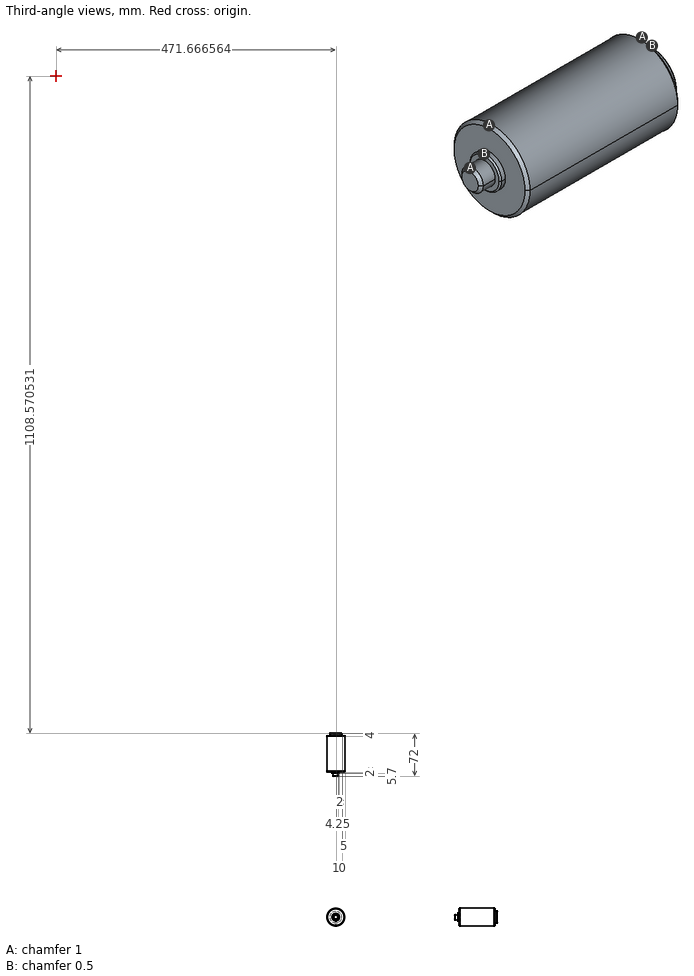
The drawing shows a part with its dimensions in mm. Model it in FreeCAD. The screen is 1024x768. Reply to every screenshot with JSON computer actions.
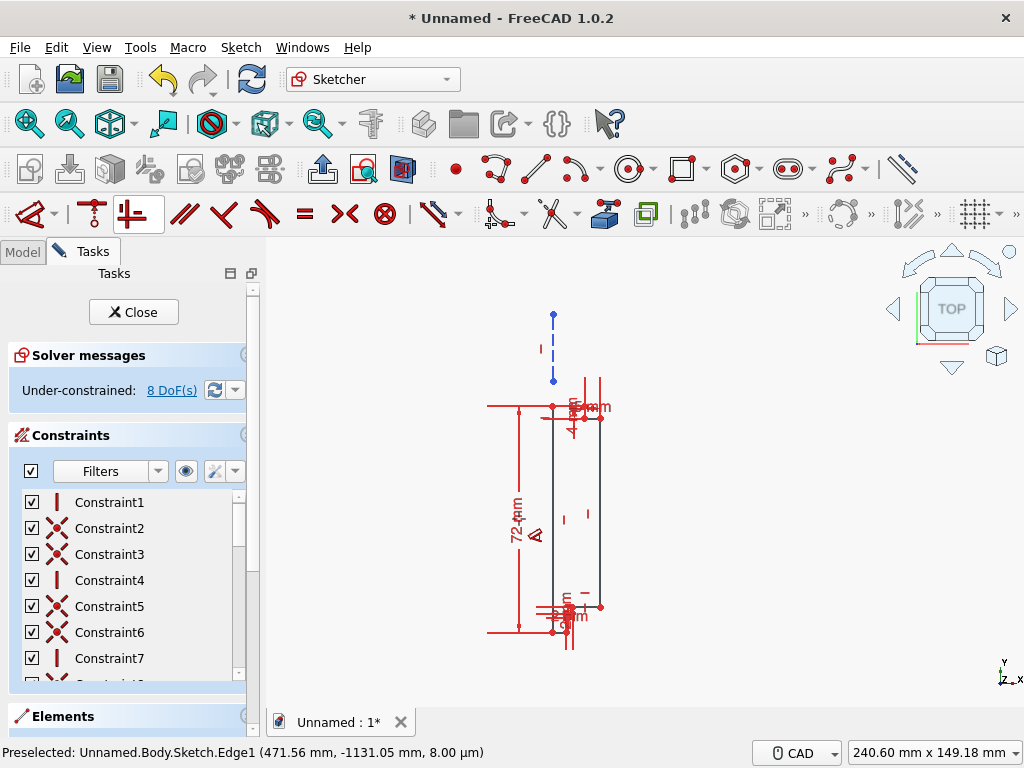
{"action": "scroll", "coordinate": [575, 406], "scroll_direction": "up", "scroll_amount": 2}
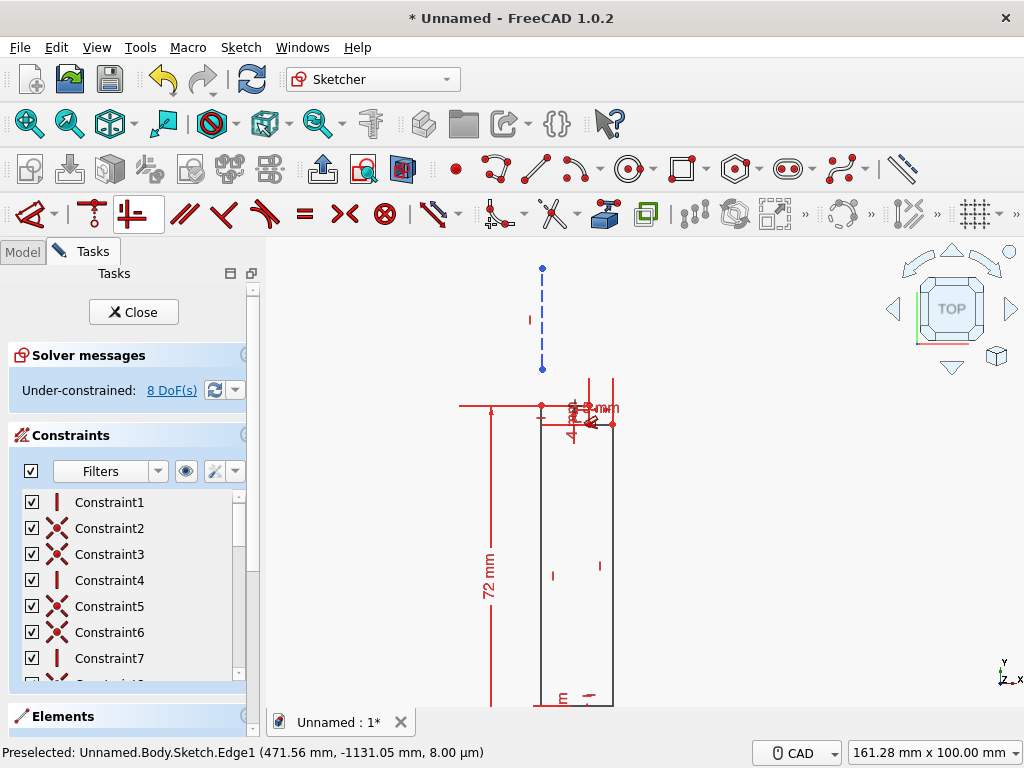
{"action": "left_click", "coordinate": [575, 406]}
{"action": "left_click", "coordinate": [565, 372]}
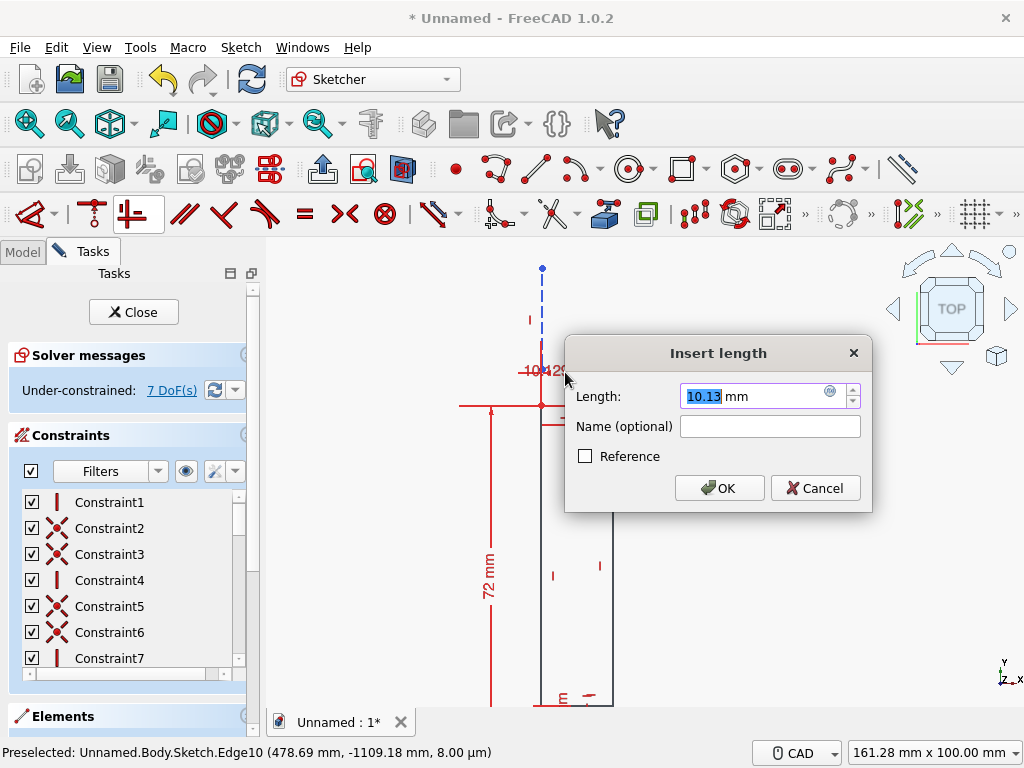
{"action": "type", "text": "10"}
{"action": "key", "text": "Return"}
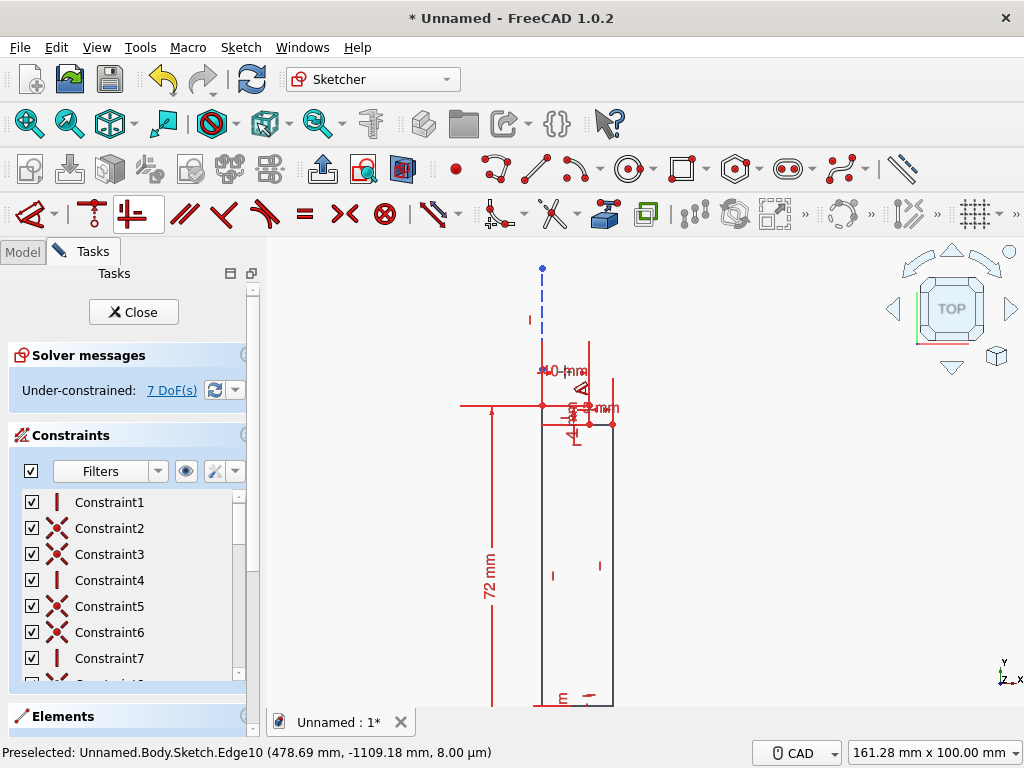
{"action": "scroll", "coordinate": [575, 406], "scroll_direction": "down", "scroll_amount": 2}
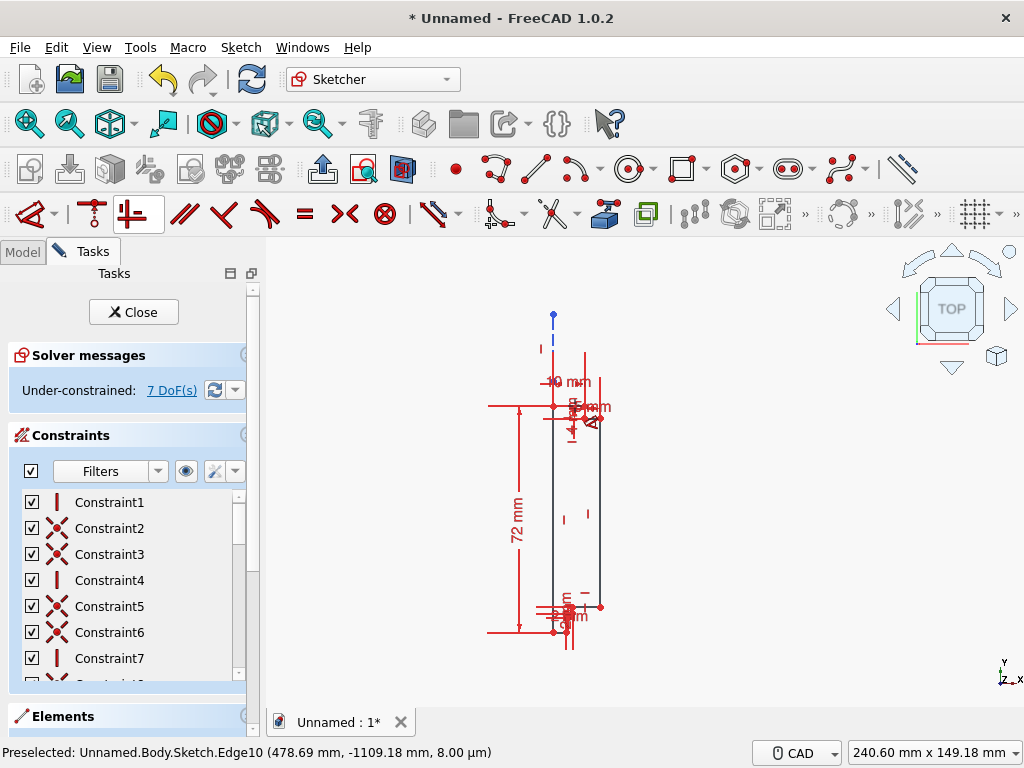
{"action": "scroll", "coordinate": [566, 625], "scroll_direction": "up", "scroll_amount": 4}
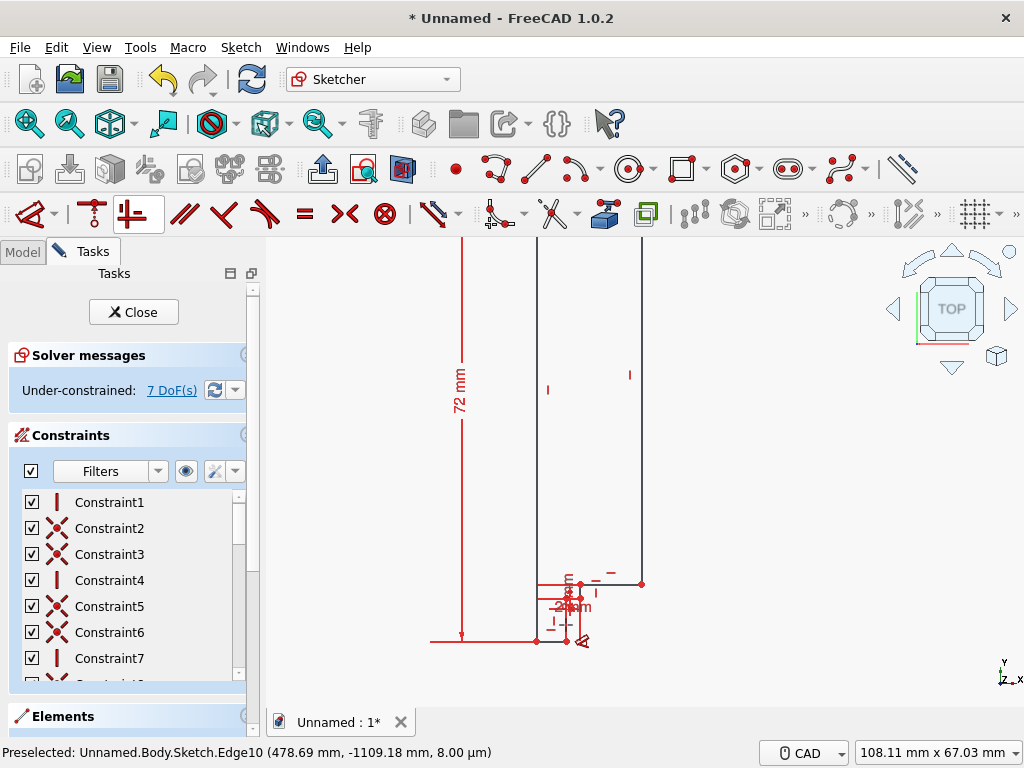
{"action": "left_click", "coordinate": [566, 624]}
{"action": "left_click", "coordinate": [600, 630]}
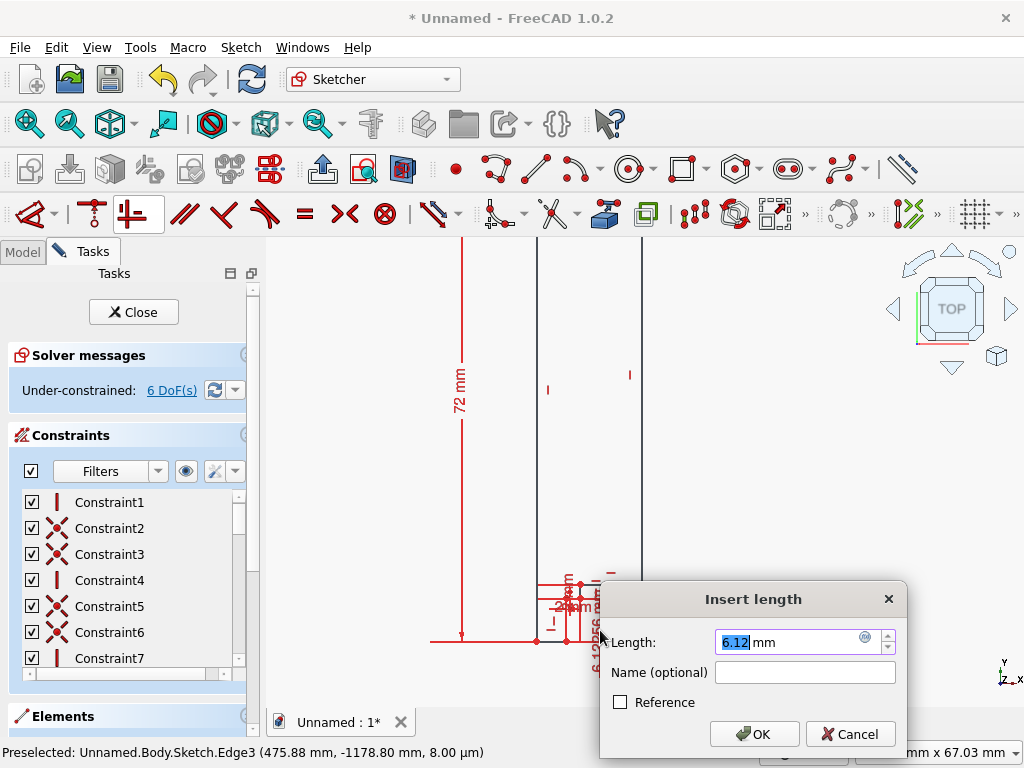
{"action": "type", "text": "5.7"}
{"action": "key", "text": "Return"}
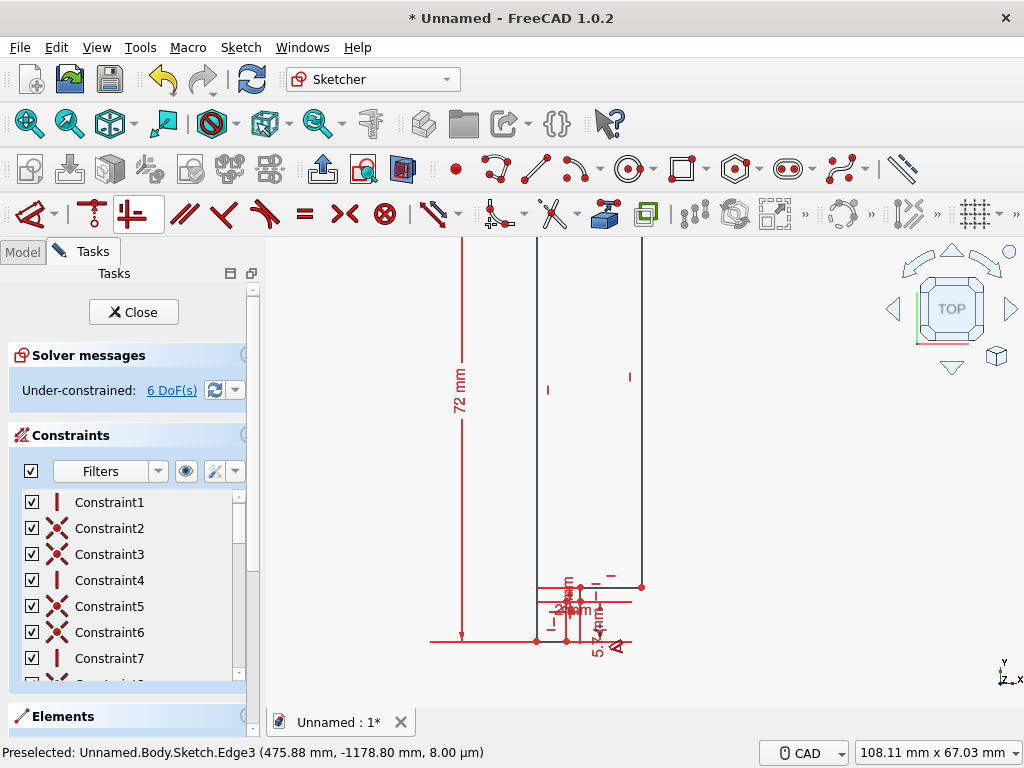
{"action": "scroll", "coordinate": [548, 642], "scroll_direction": "up", "scroll_amount": 2}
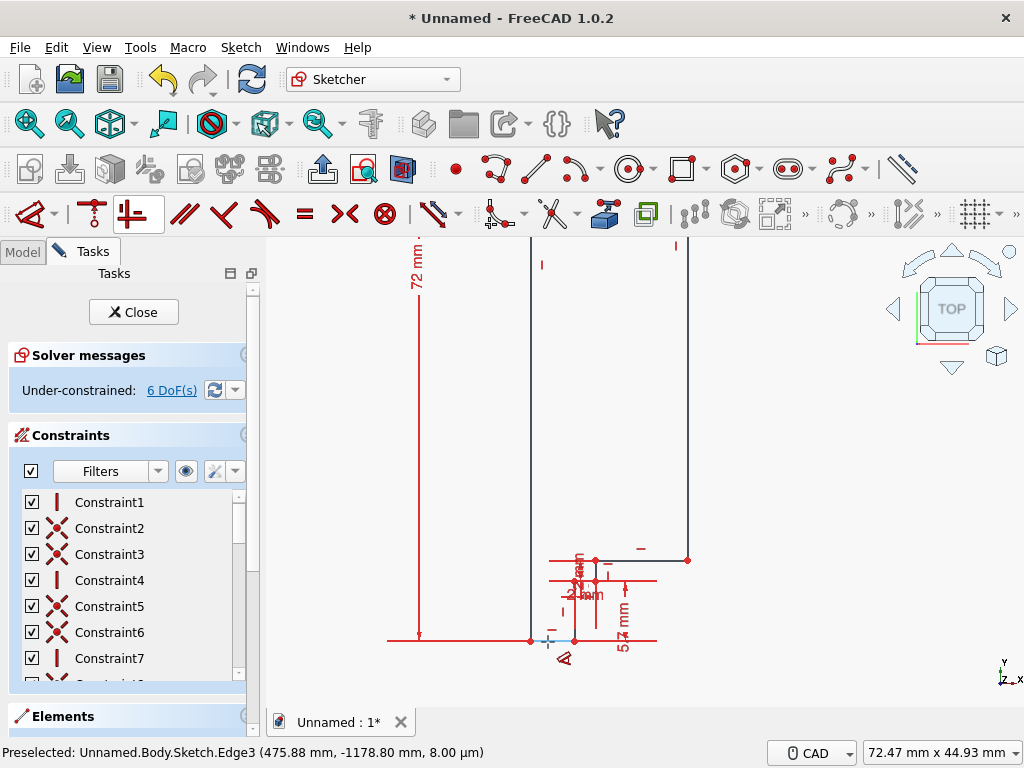
{"action": "left_click", "coordinate": [549, 641]}
{"action": "left_click", "coordinate": [553, 675]}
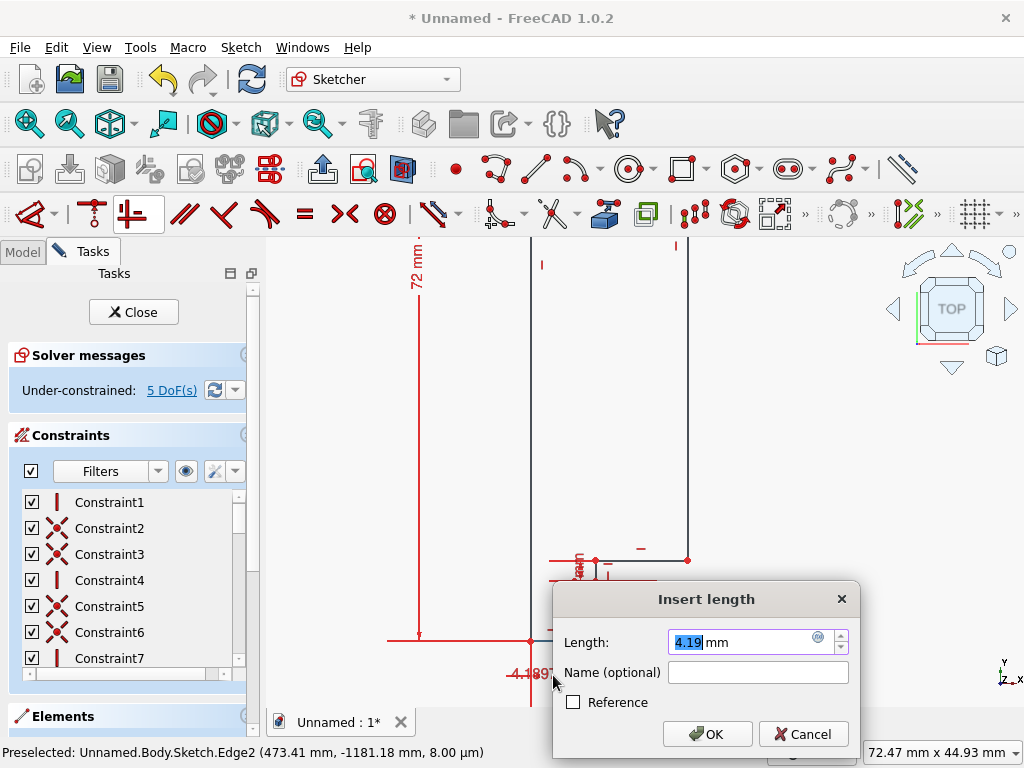
{"action": "type", "text": "4.25"}
{"action": "key", "text": "Return"}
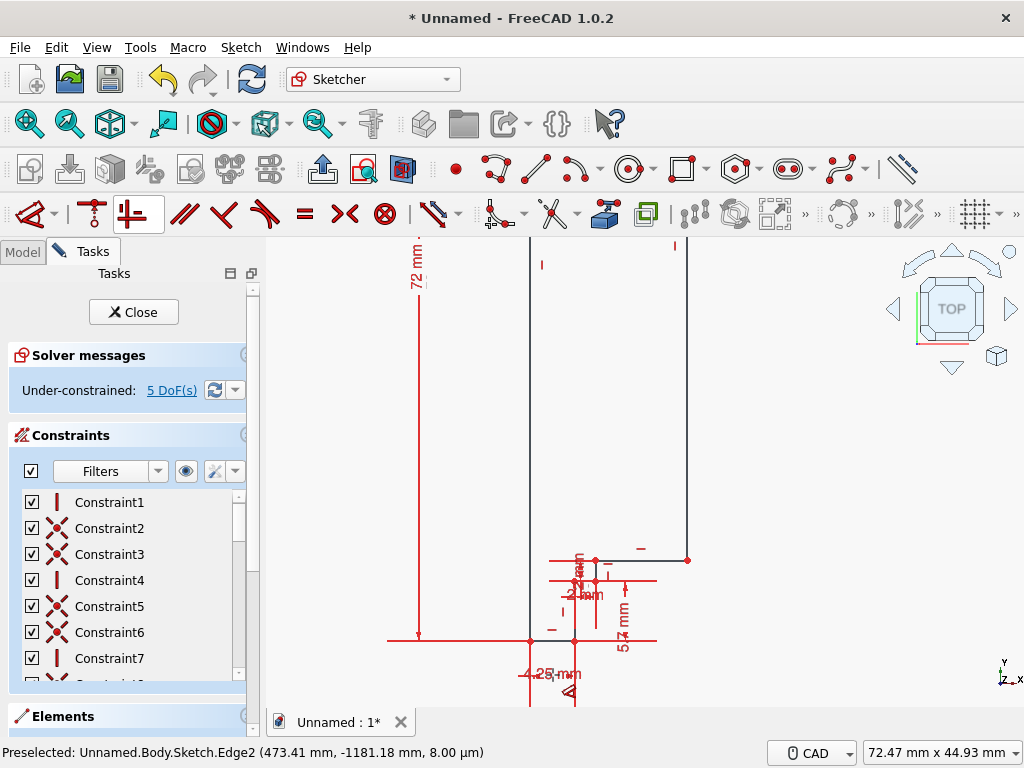
{"action": "scroll", "coordinate": [562, 629], "scroll_direction": "down", "scroll_amount": 6}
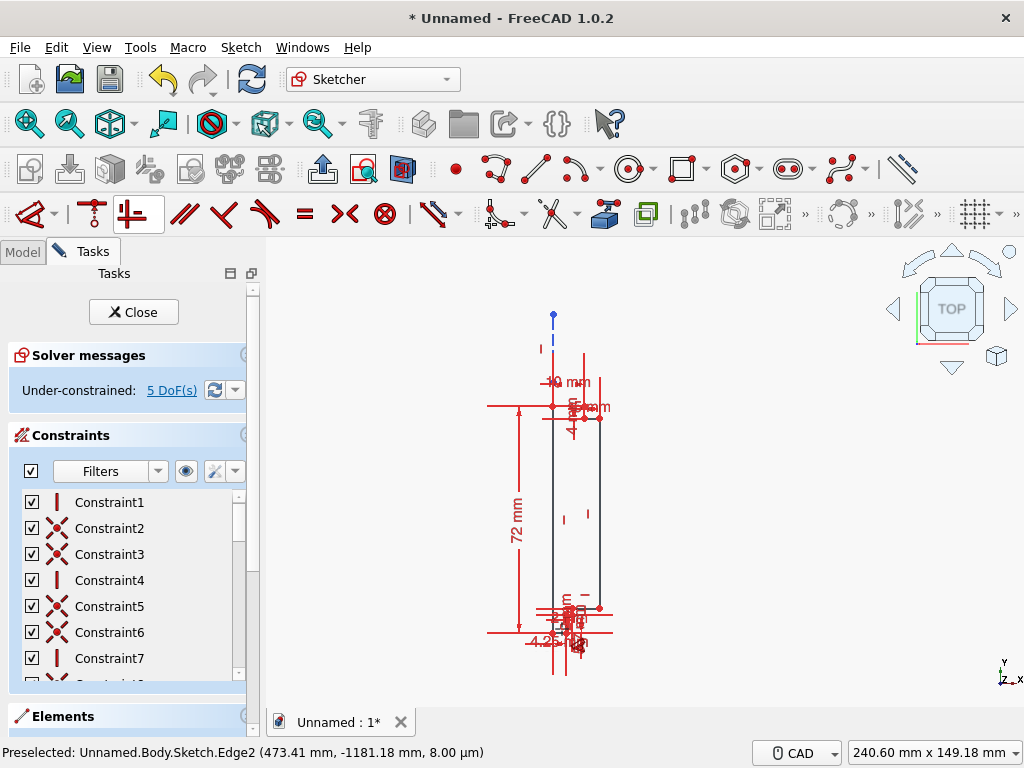
{"action": "left_click", "coordinate": [553, 406]}
{"action": "left_click", "coordinate": [423, 440]}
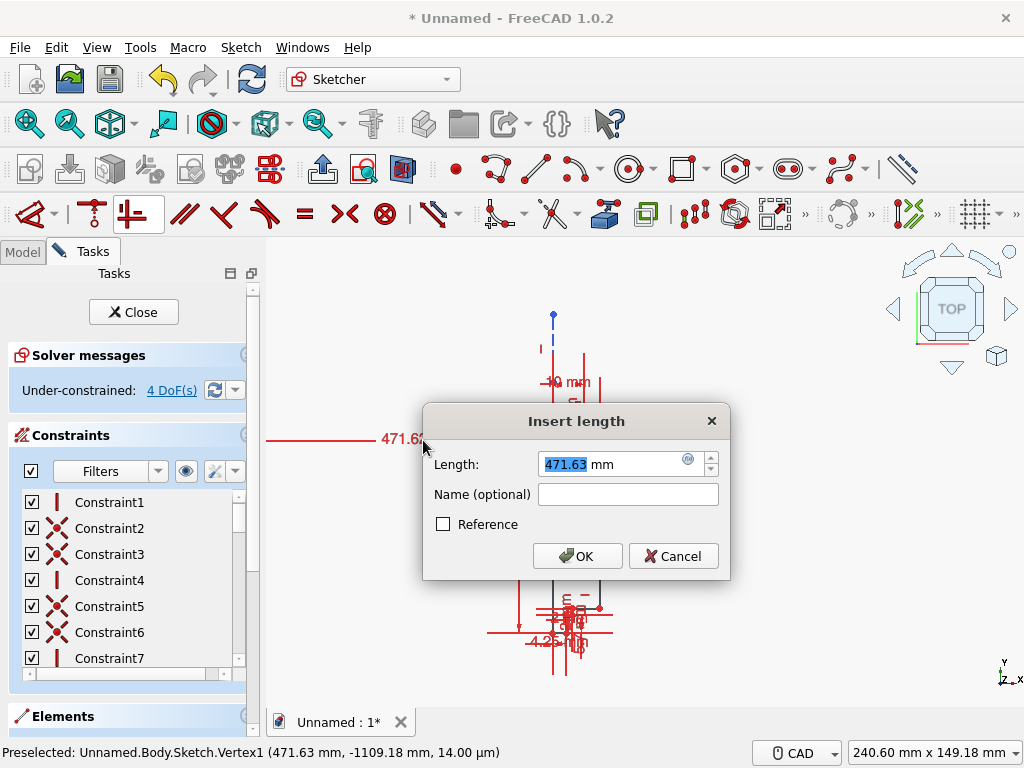
{"action": "type", "text": "471.666564"}
{"action": "key", "text": "Return"}